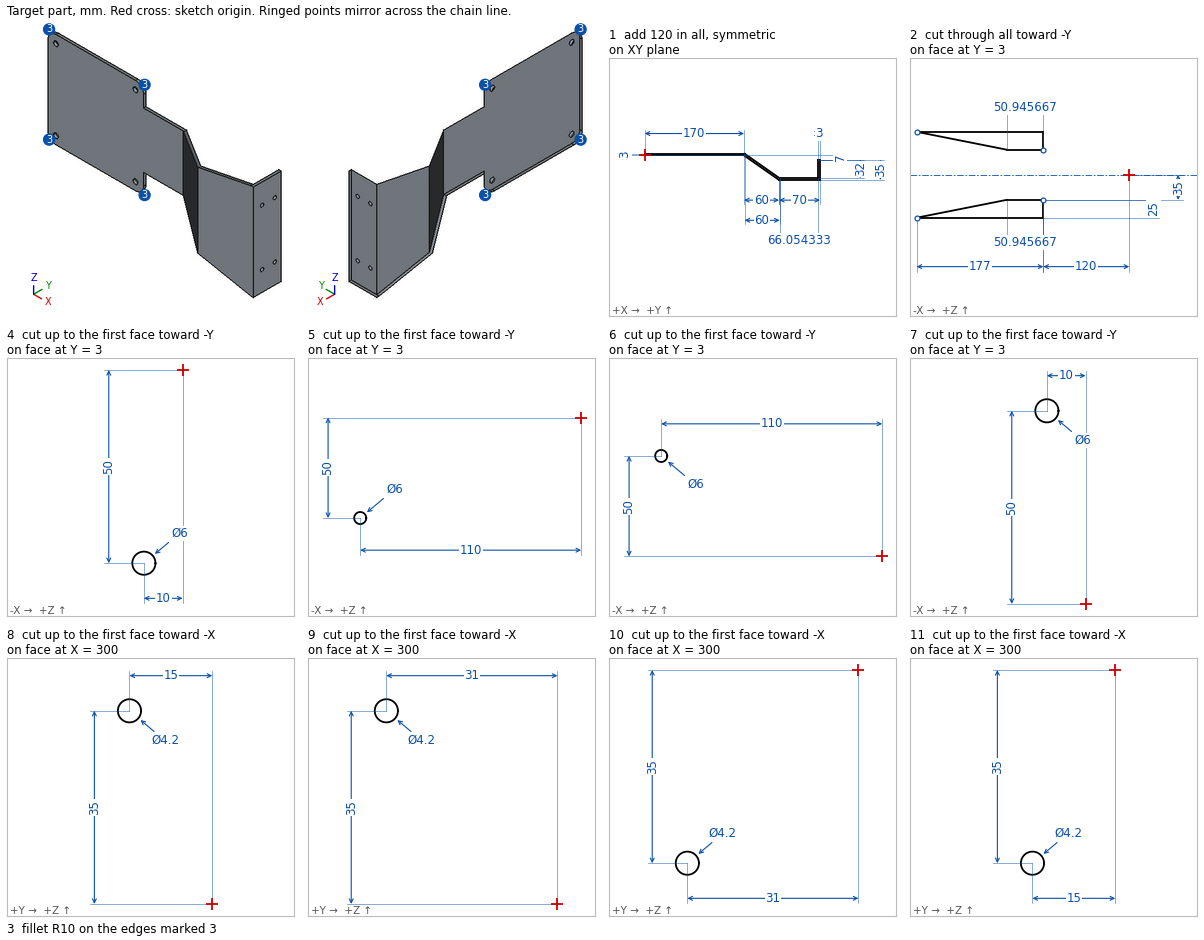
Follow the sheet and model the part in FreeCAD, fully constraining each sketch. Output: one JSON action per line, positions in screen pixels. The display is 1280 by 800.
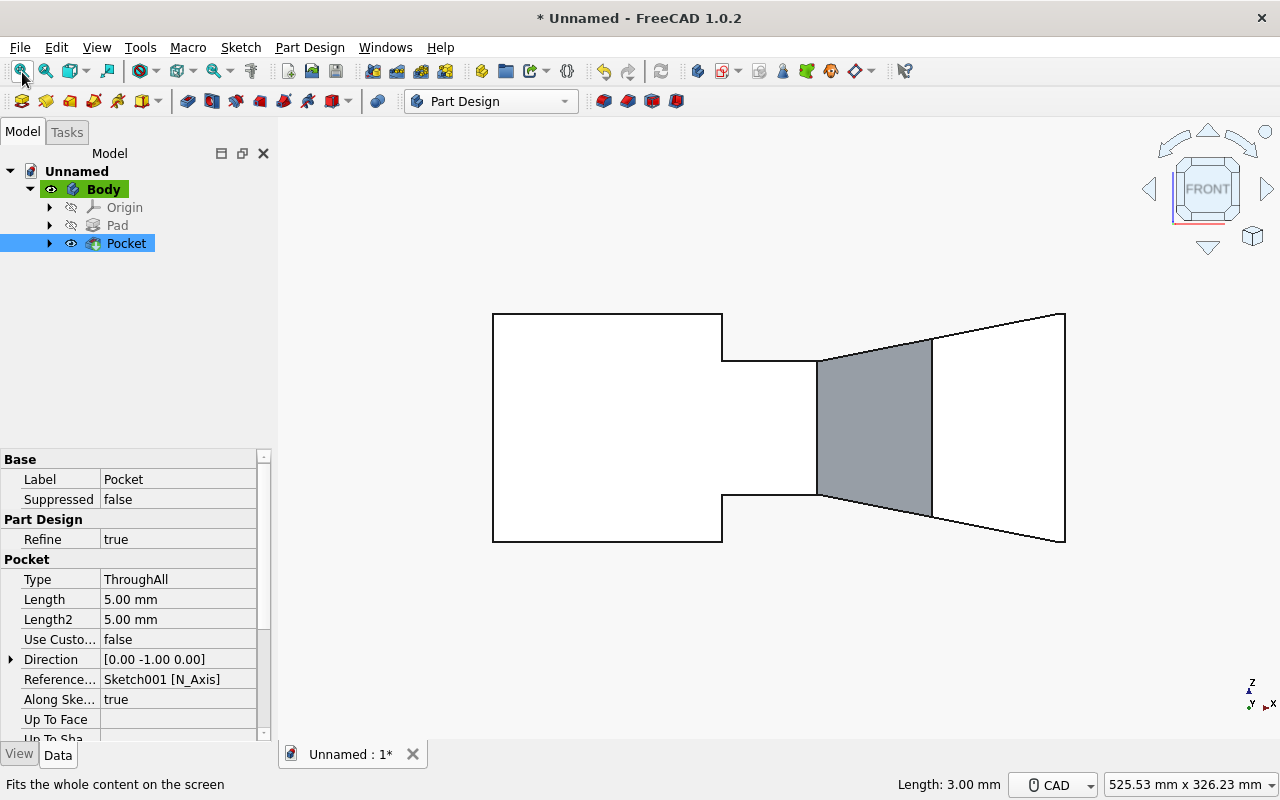
{"action": "key", "text": "3"}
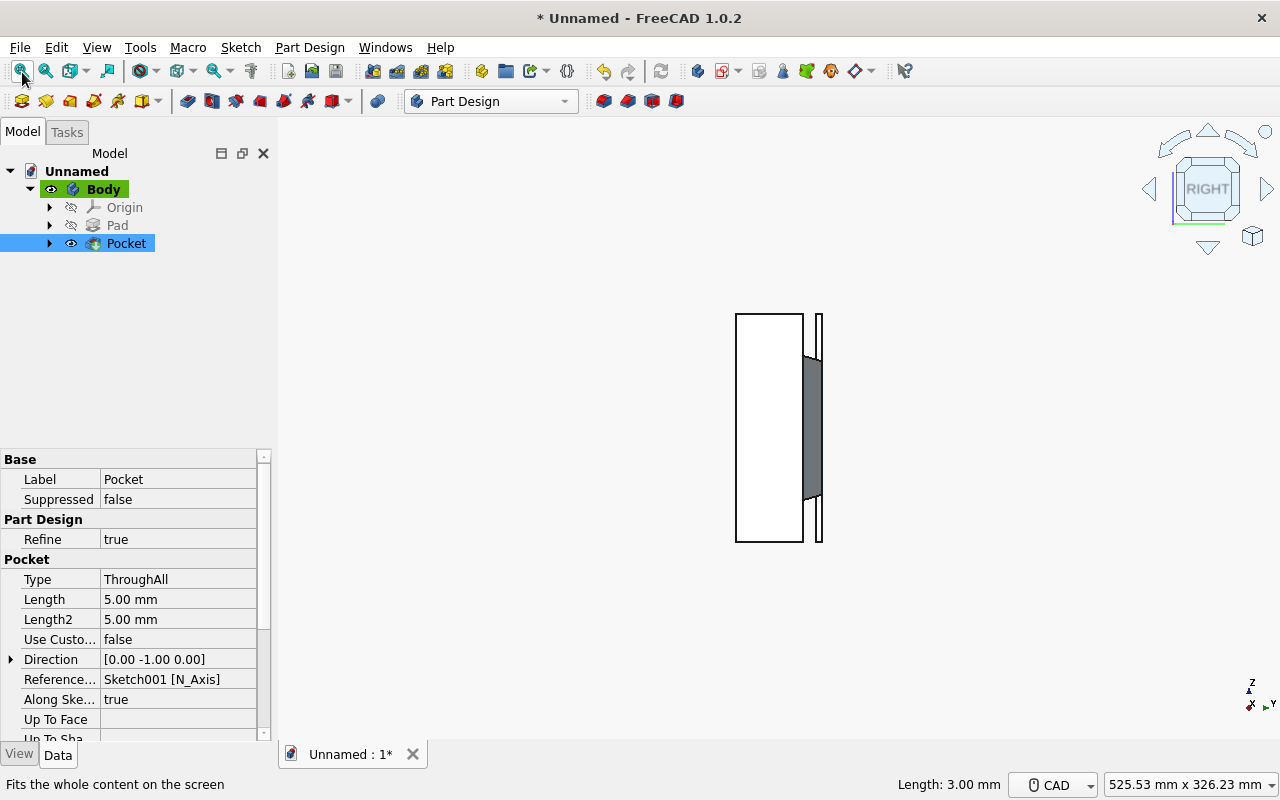
{"action": "left_click", "coordinate": [22, 72]}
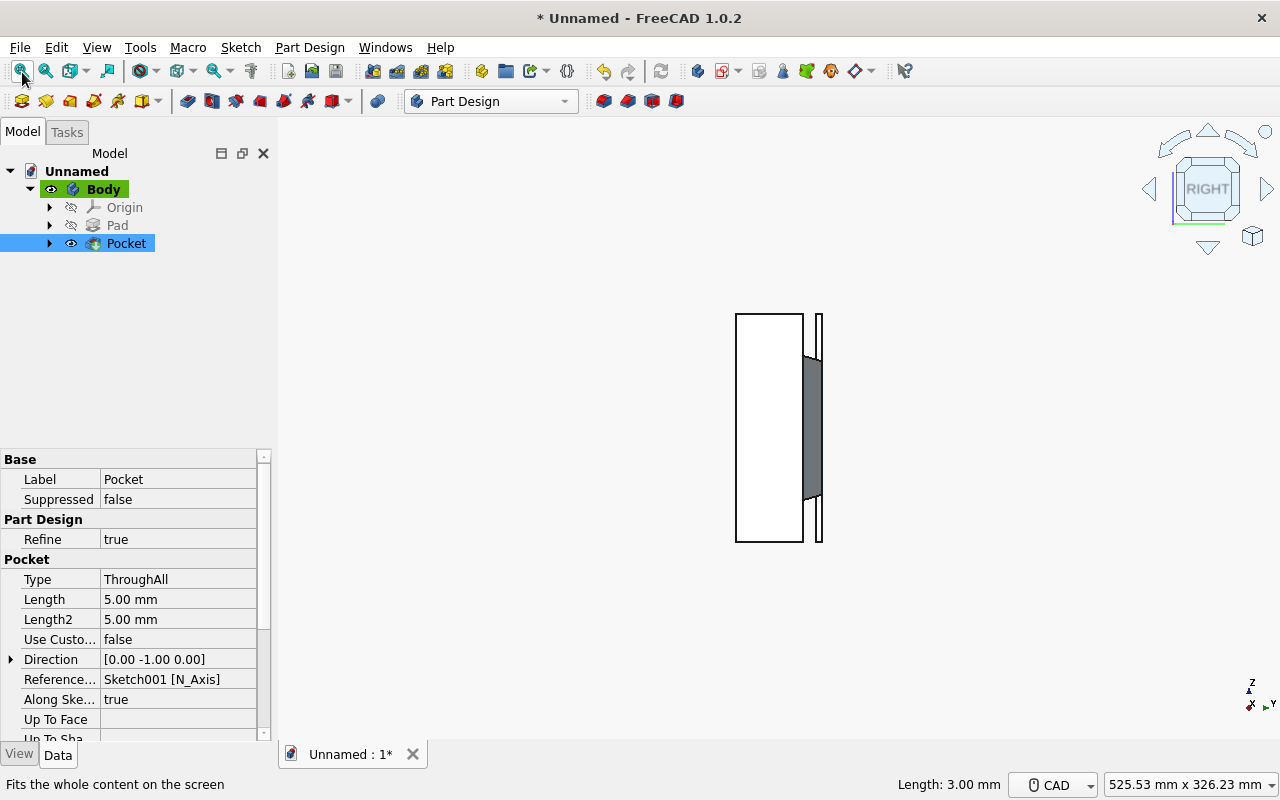
{"action": "scroll", "coordinate": [819, 541], "scroll_direction": "up", "scroll_amount": 10}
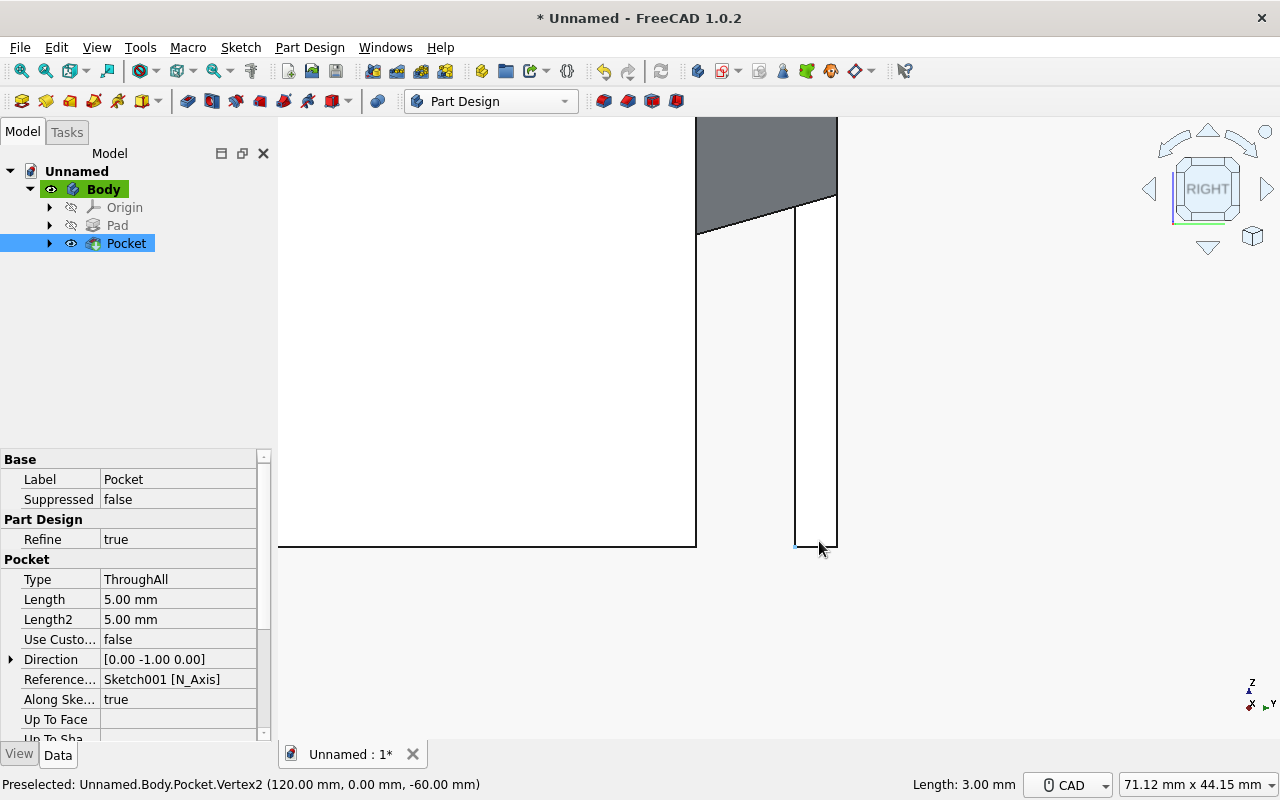
{"action": "left_click", "coordinate": [816, 546], "text": "ctrl"}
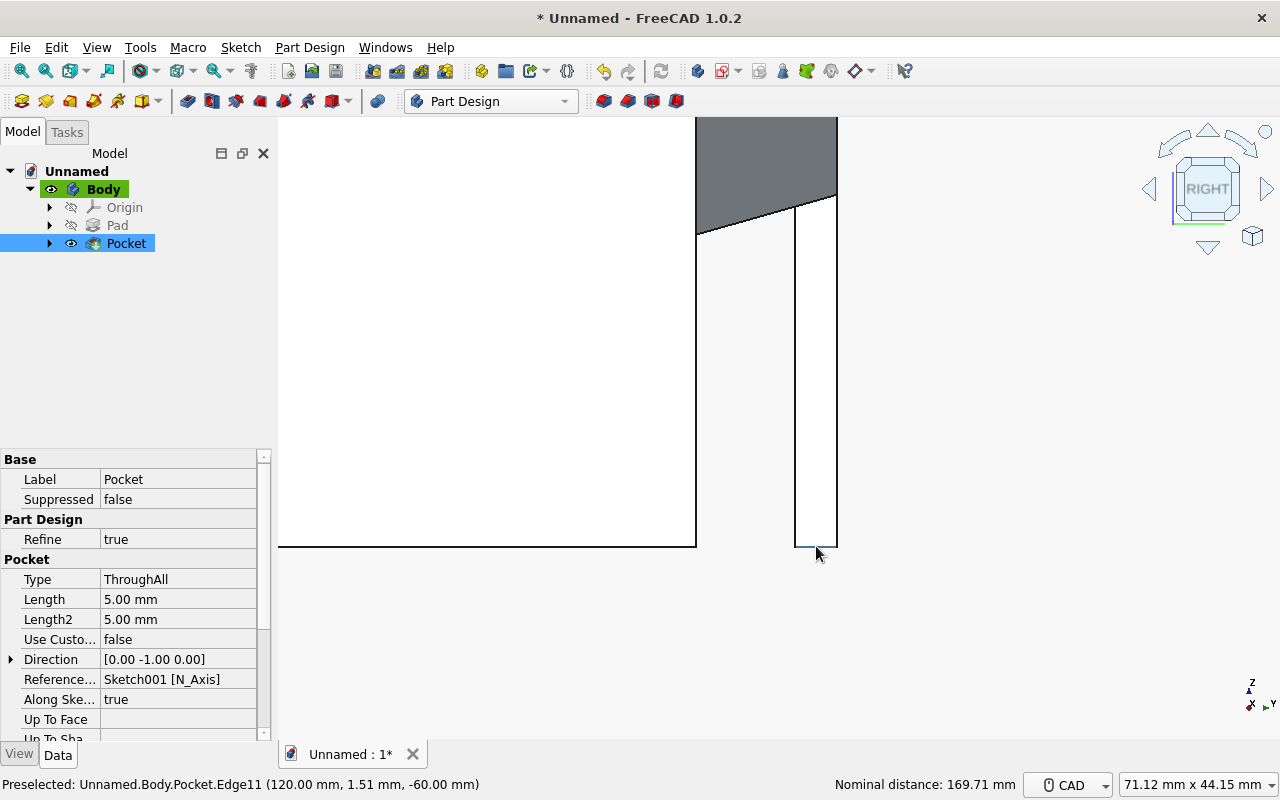
{"action": "left_click", "coordinate": [22, 72]}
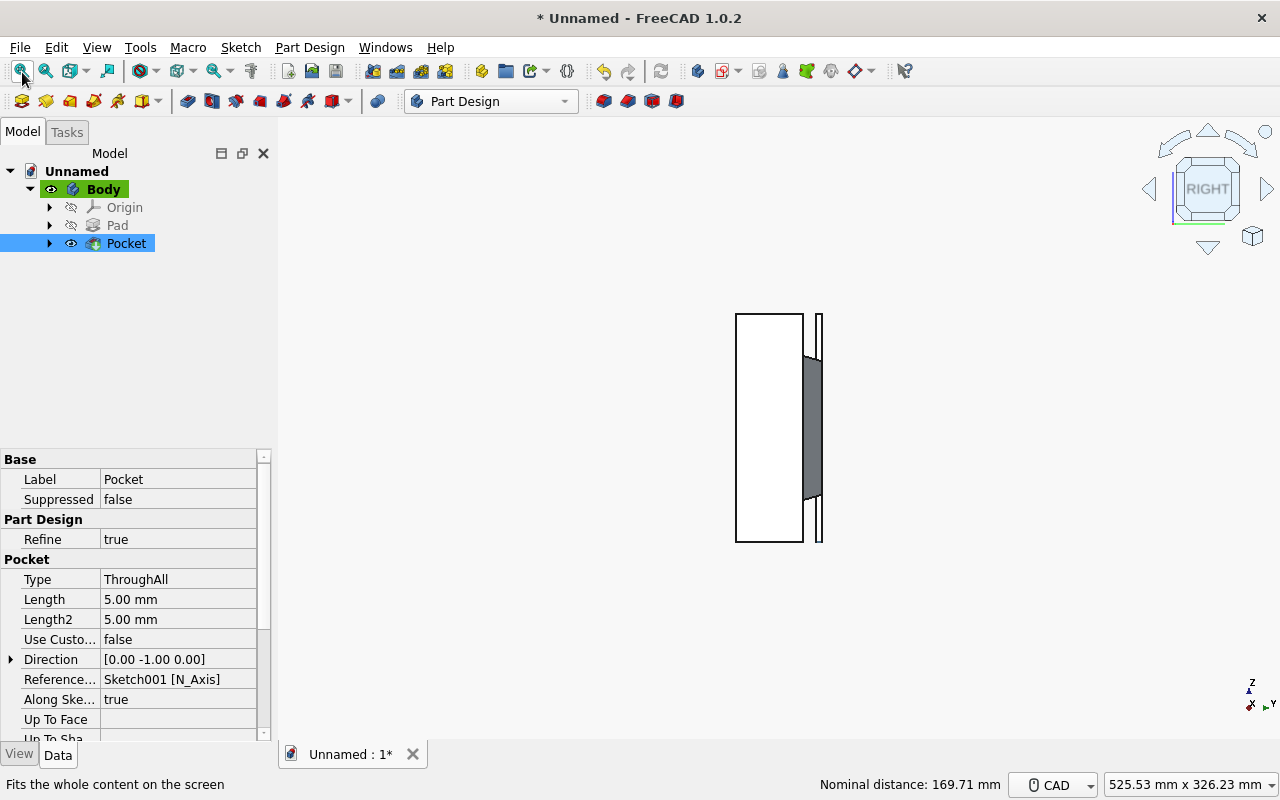
{"action": "key", "text": "5"}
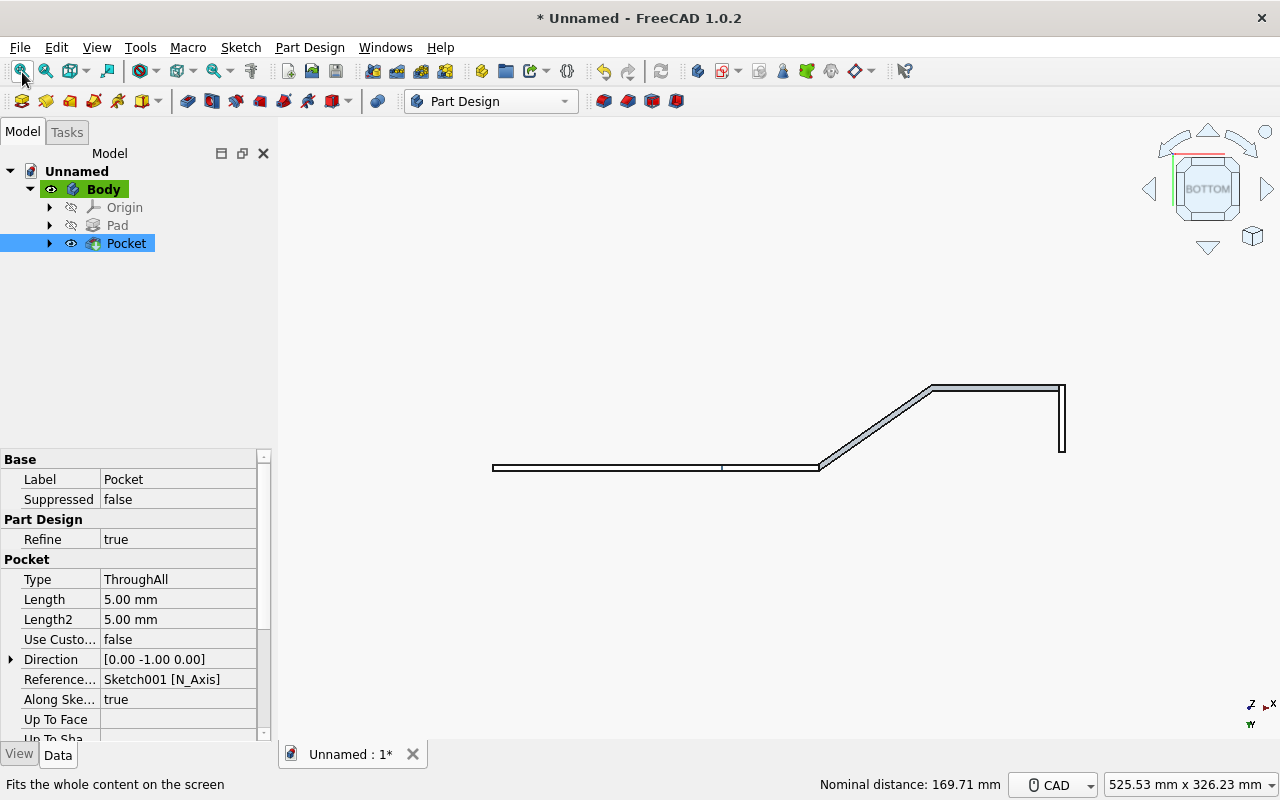
{"action": "scroll", "coordinate": [493, 467], "scroll_direction": "up", "scroll_amount": 10}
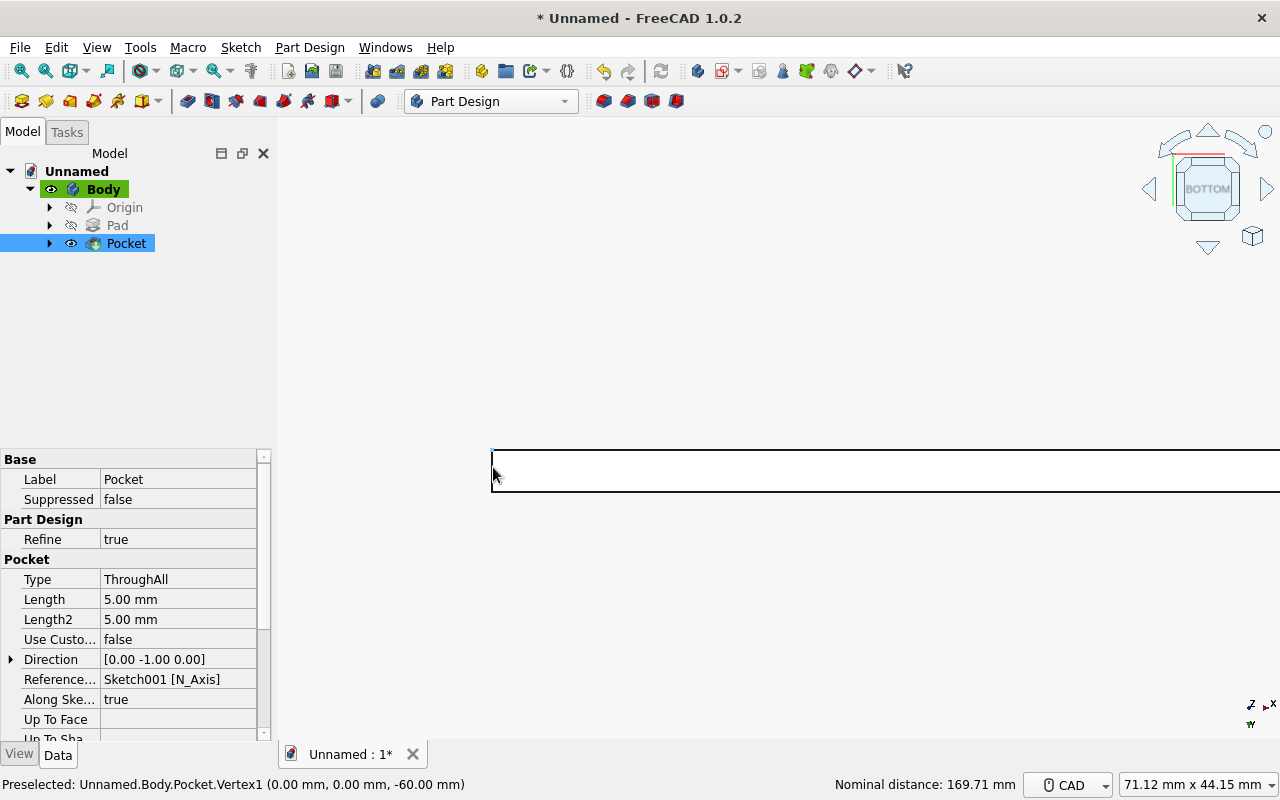
{"action": "left_click", "coordinate": [492, 470], "text": "ctrl"}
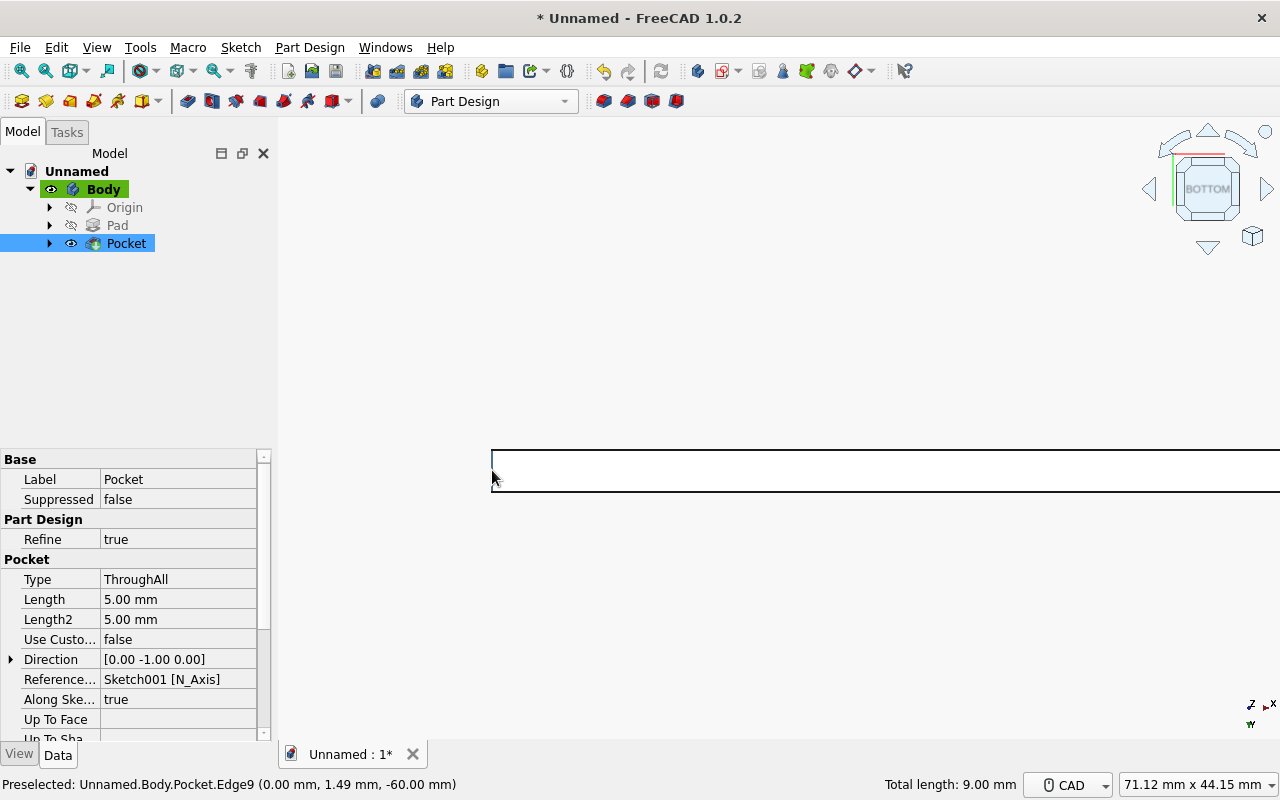
{"action": "left_click", "coordinate": [22, 72]}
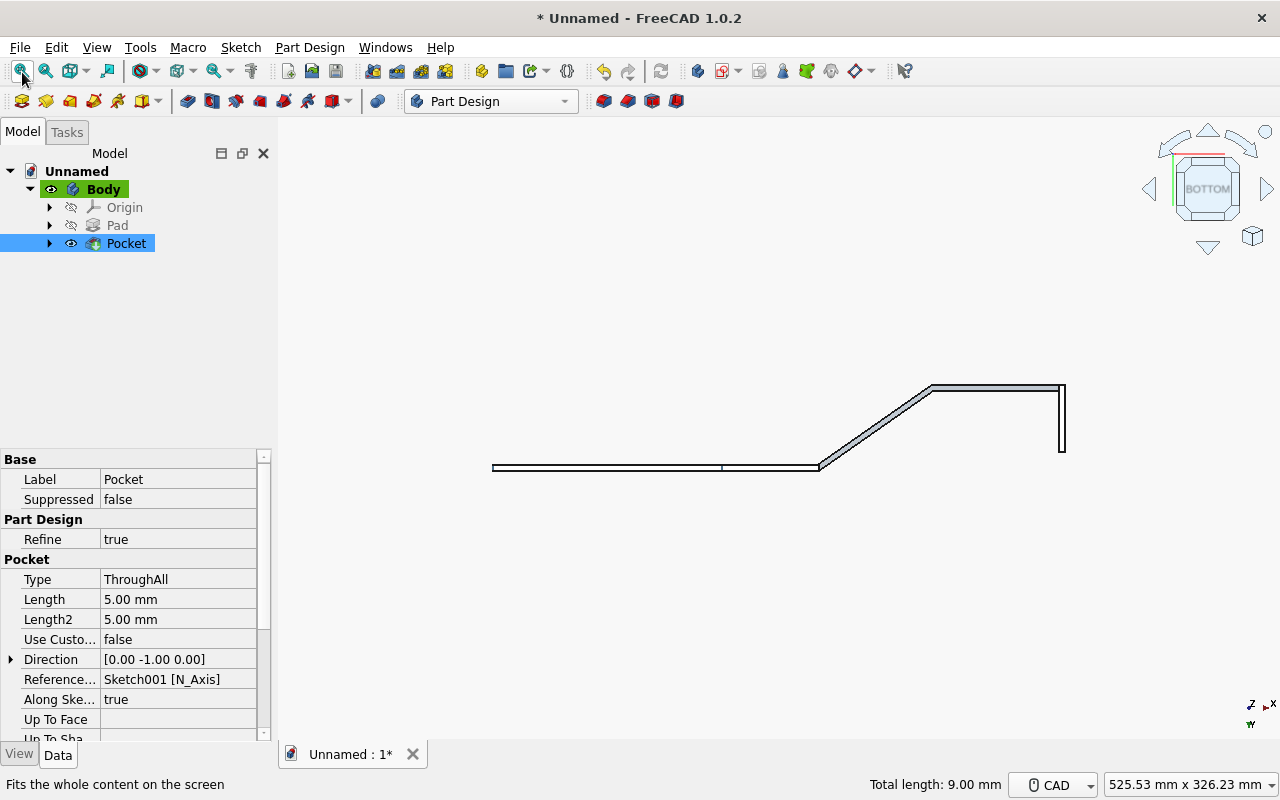
{"action": "key", "text": "4"}